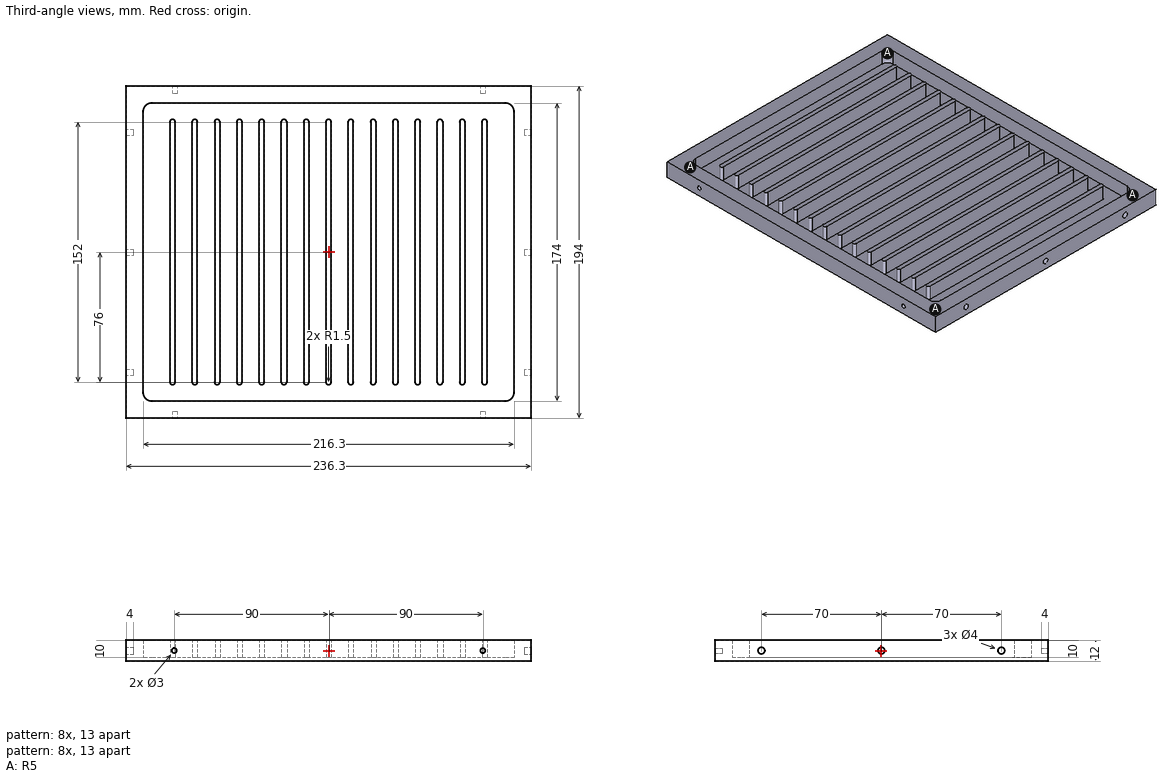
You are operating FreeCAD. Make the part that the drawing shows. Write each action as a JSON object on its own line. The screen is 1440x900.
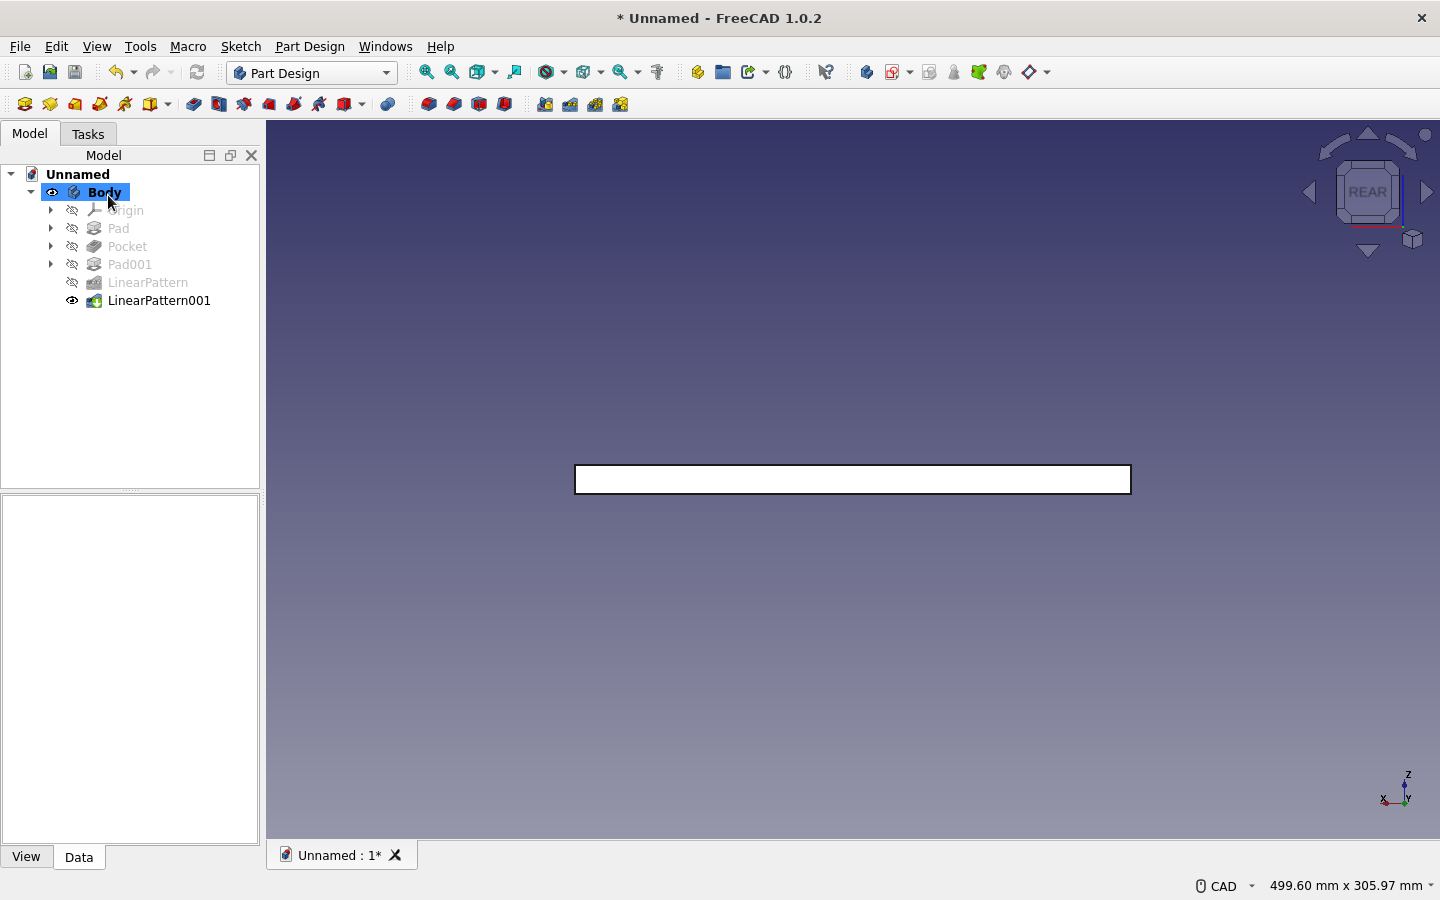
{"action": "left_click", "coordinate": [615, 478]}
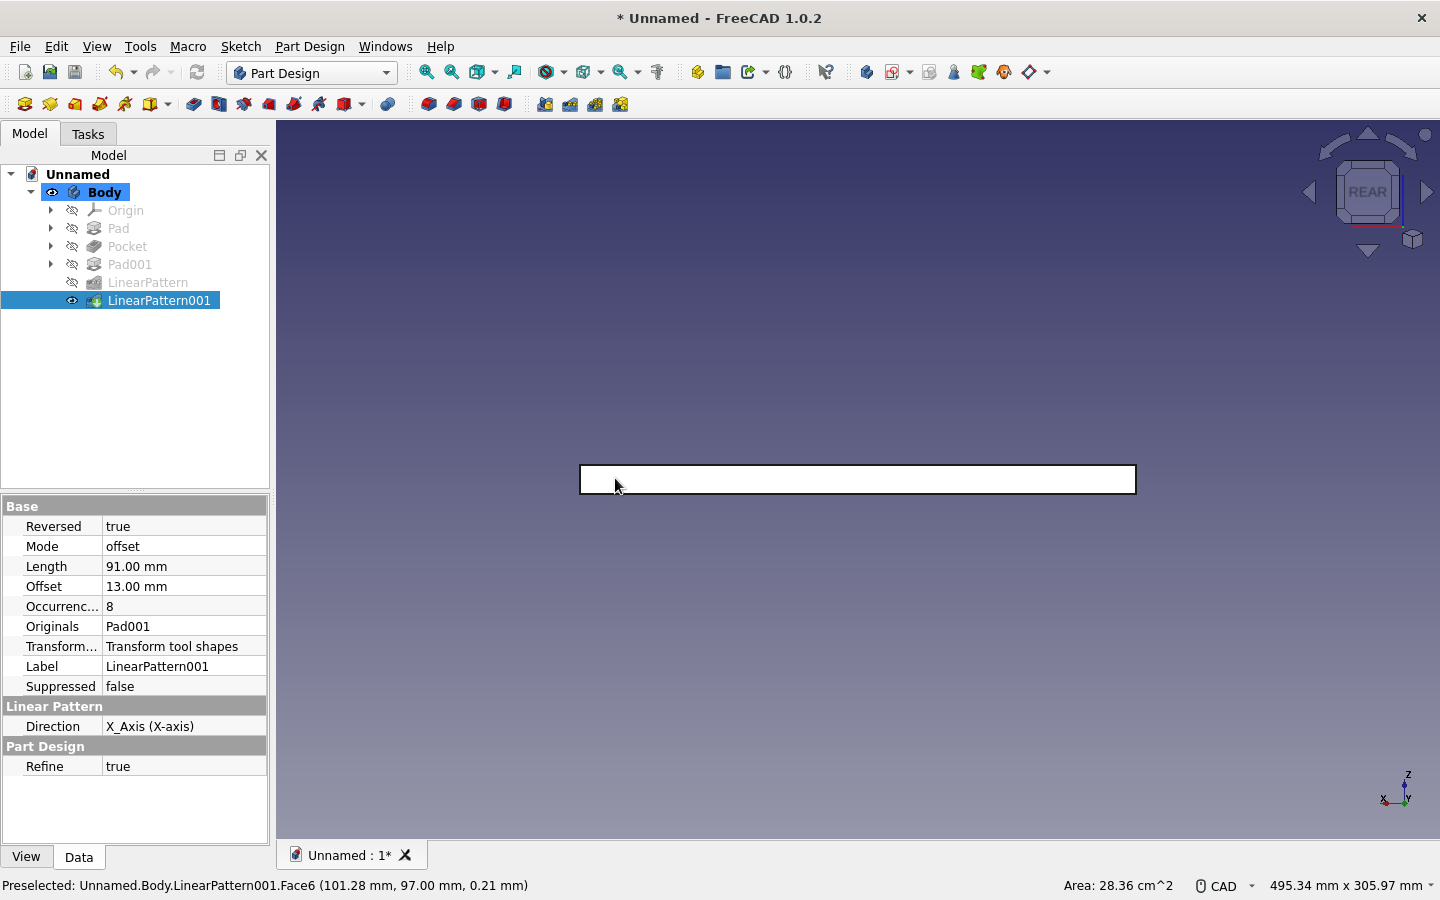
{"action": "left_click", "coordinate": [892, 72]}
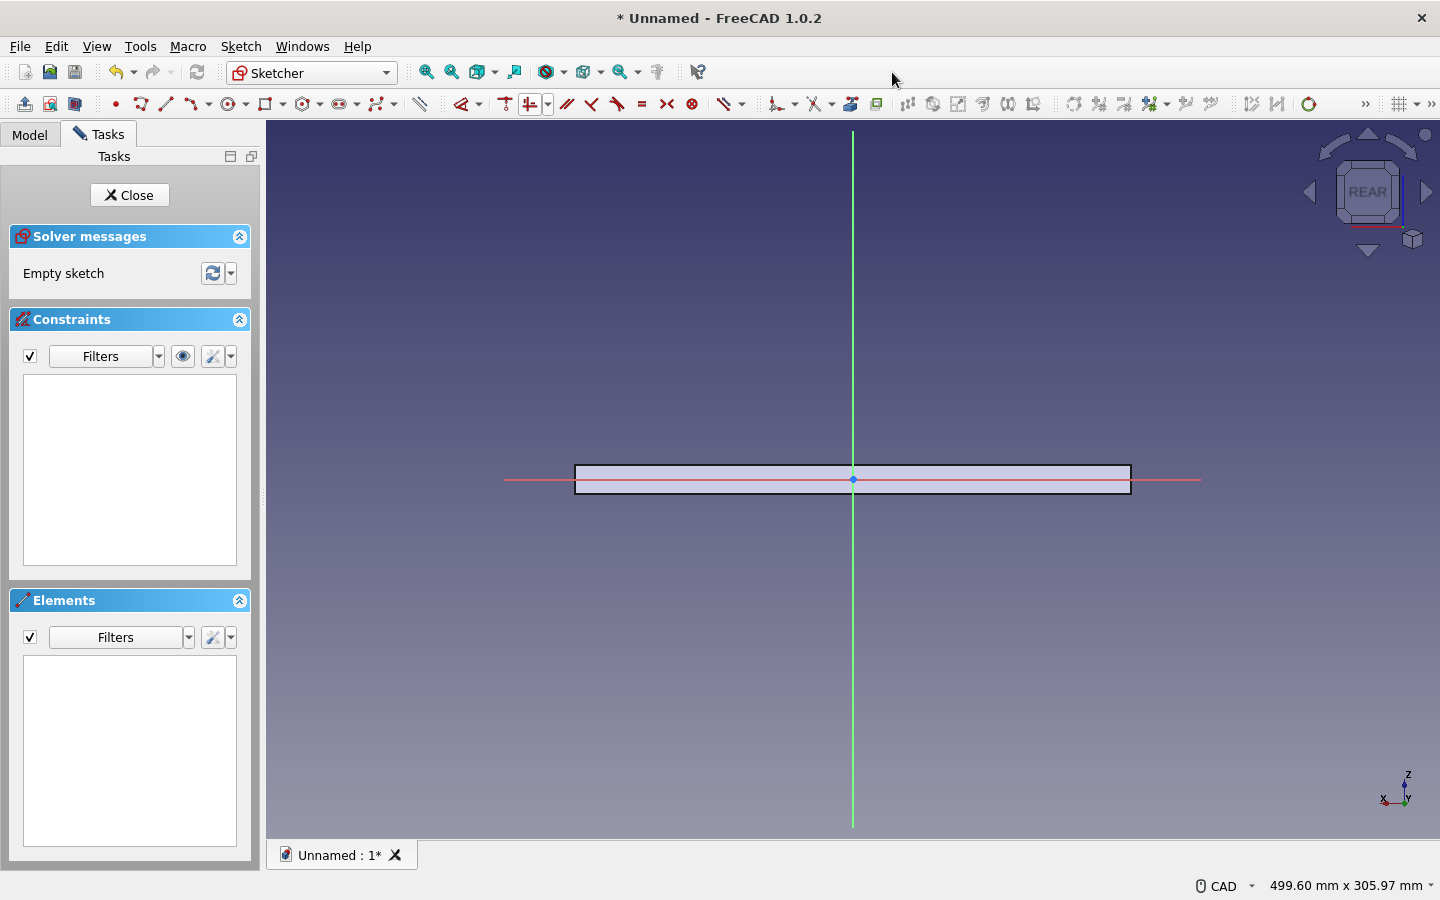
{"action": "scroll", "coordinate": [992, 479], "scroll_direction": "up", "scroll_amount": 2}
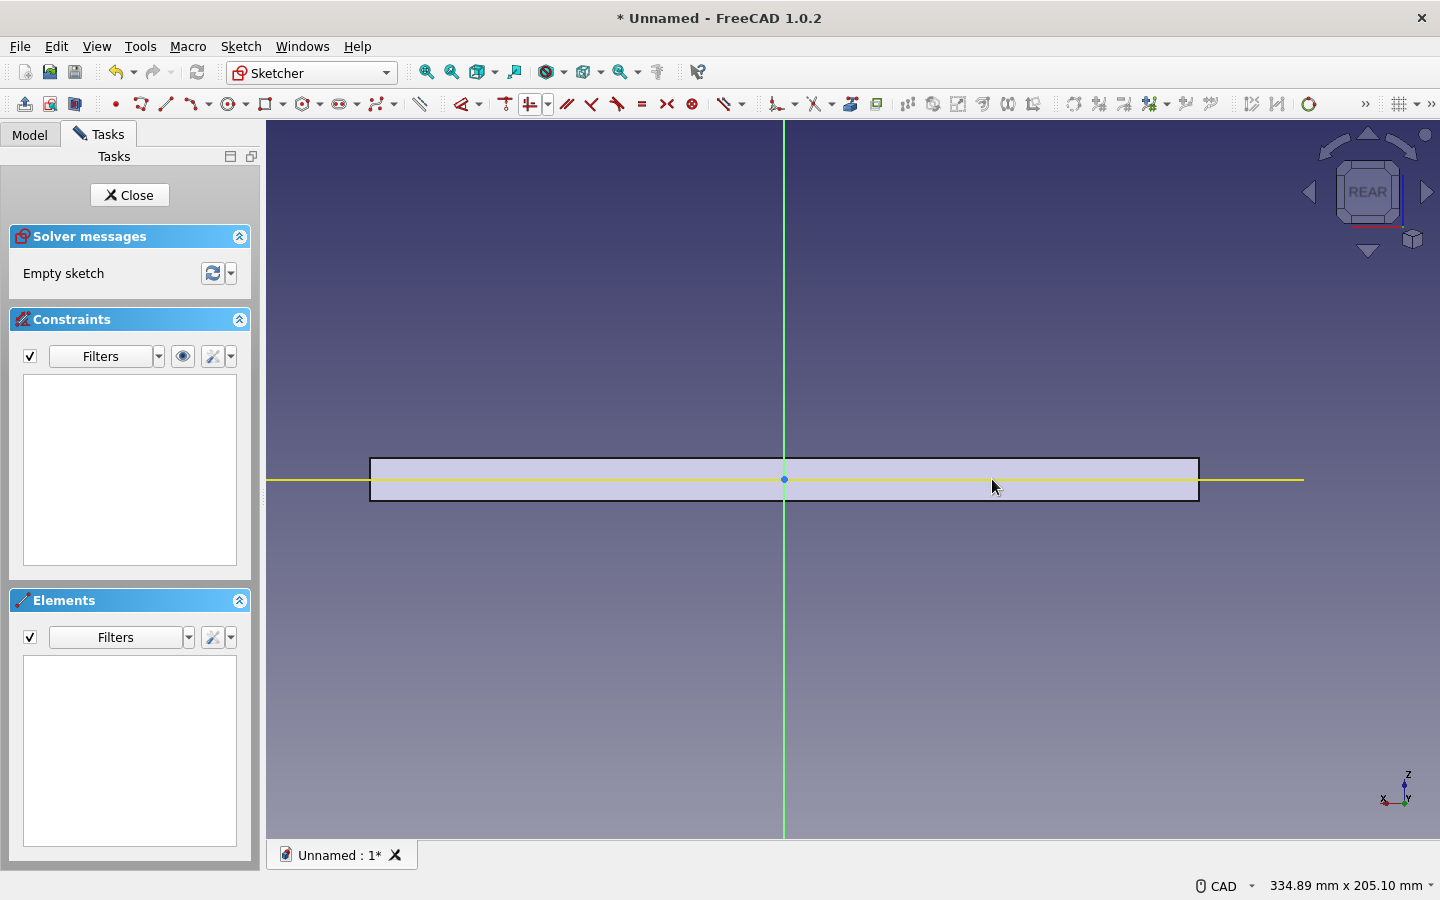
{"action": "left_click", "coordinate": [228, 104]}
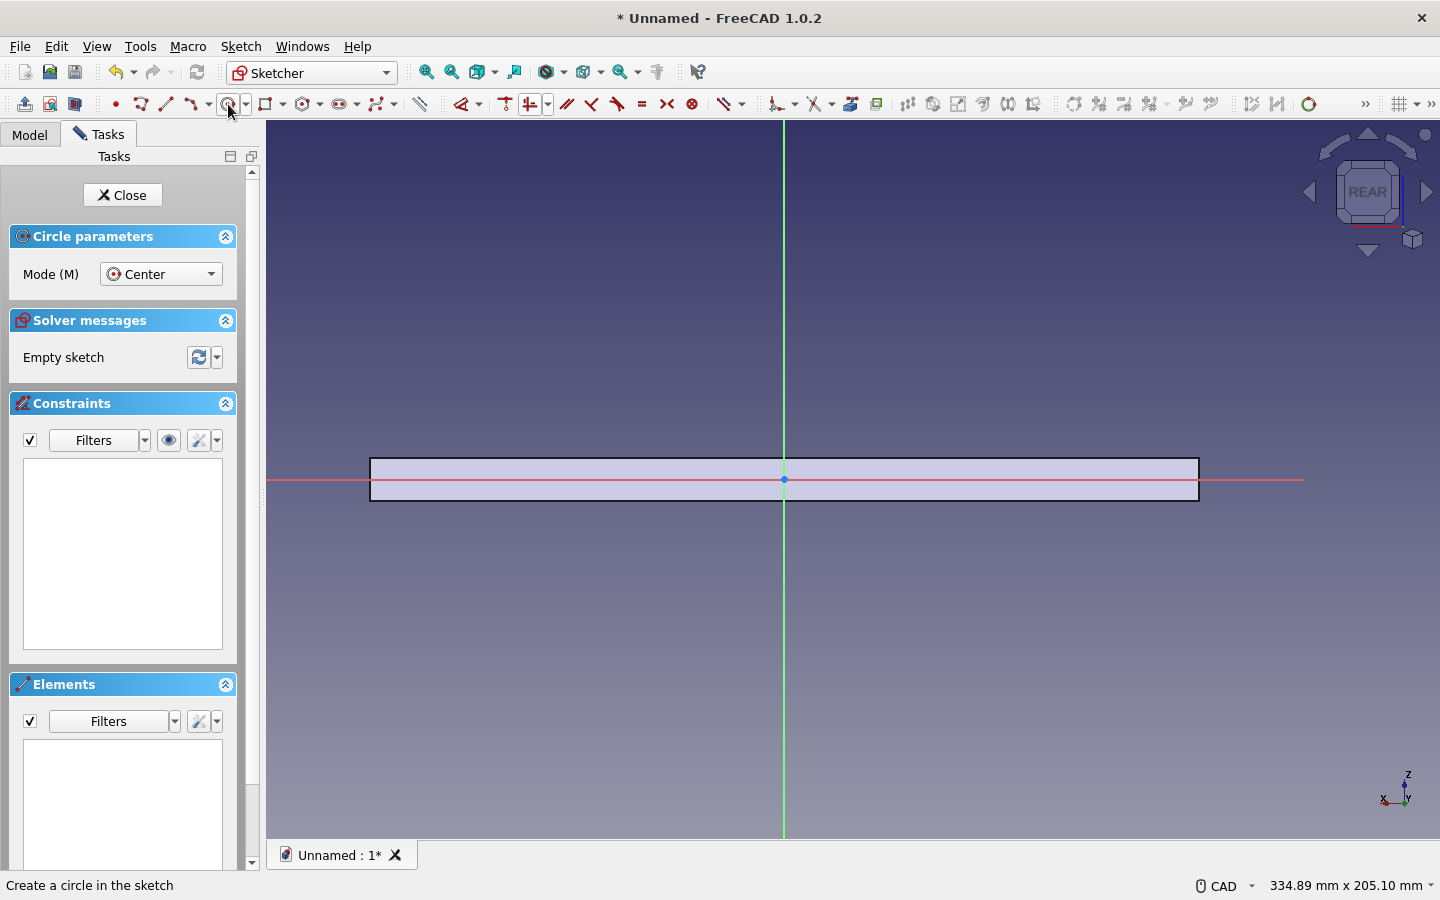
{"action": "scroll", "coordinate": [1100, 479], "scroll_direction": "up", "scroll_amount": 8}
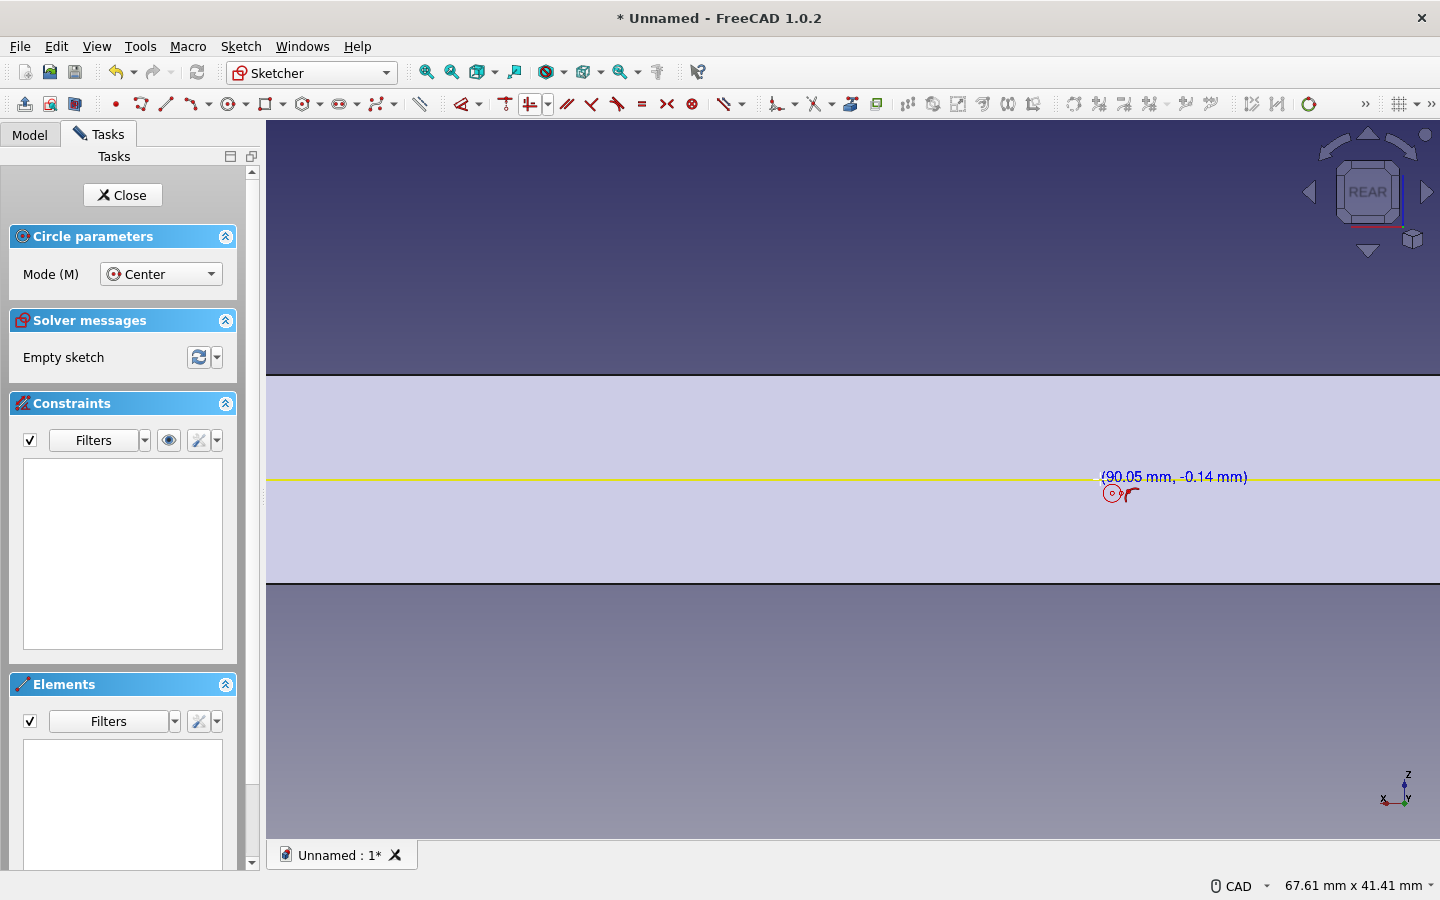
{"action": "scroll", "coordinate": [1101, 480], "scroll_direction": "down", "scroll_amount": 8}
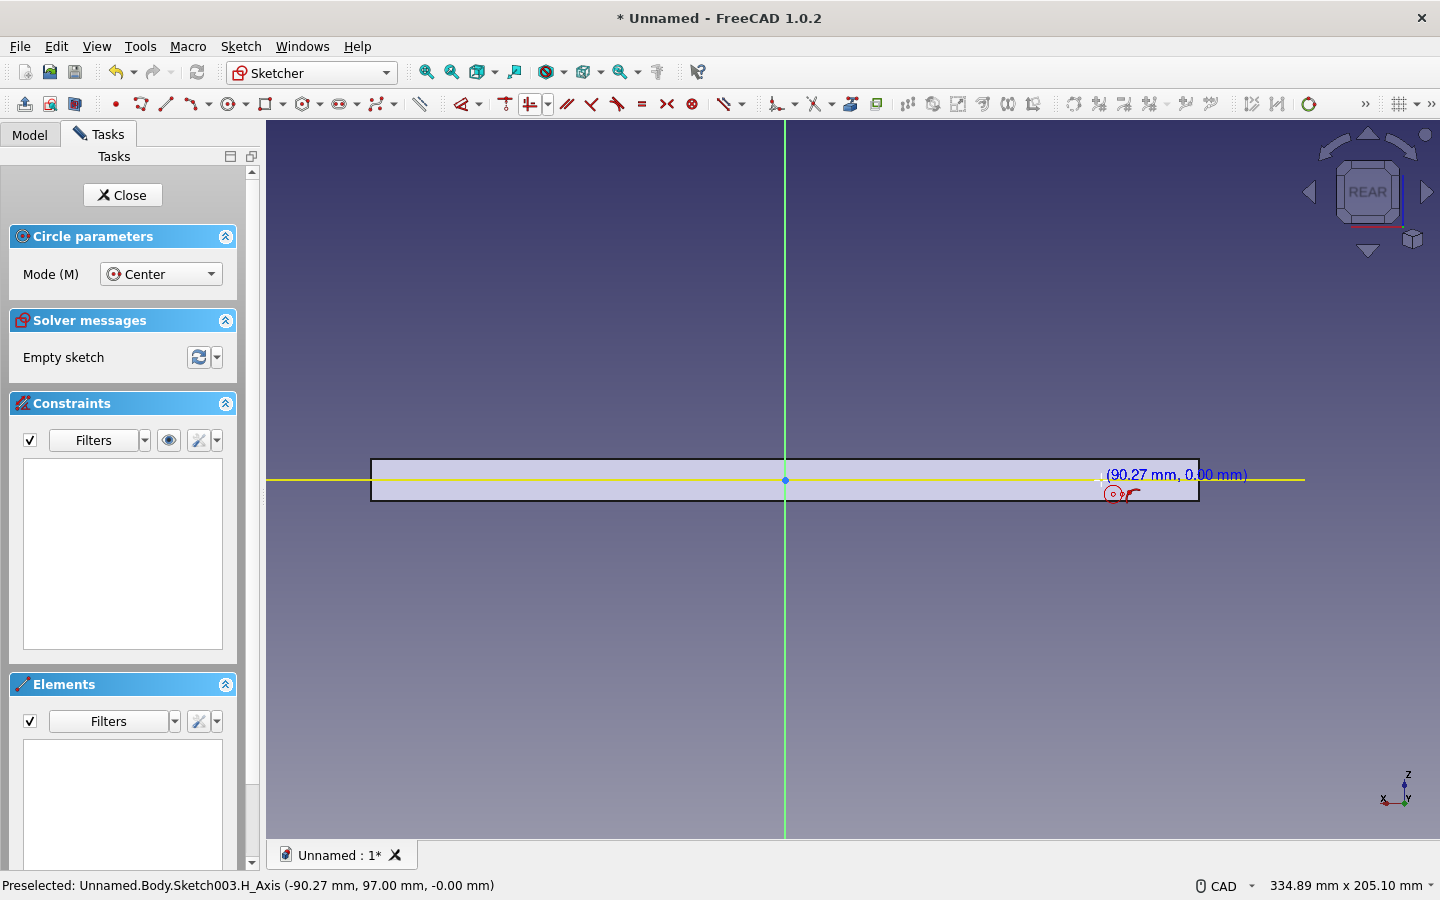
{"action": "left_click", "coordinate": [1101, 480]}